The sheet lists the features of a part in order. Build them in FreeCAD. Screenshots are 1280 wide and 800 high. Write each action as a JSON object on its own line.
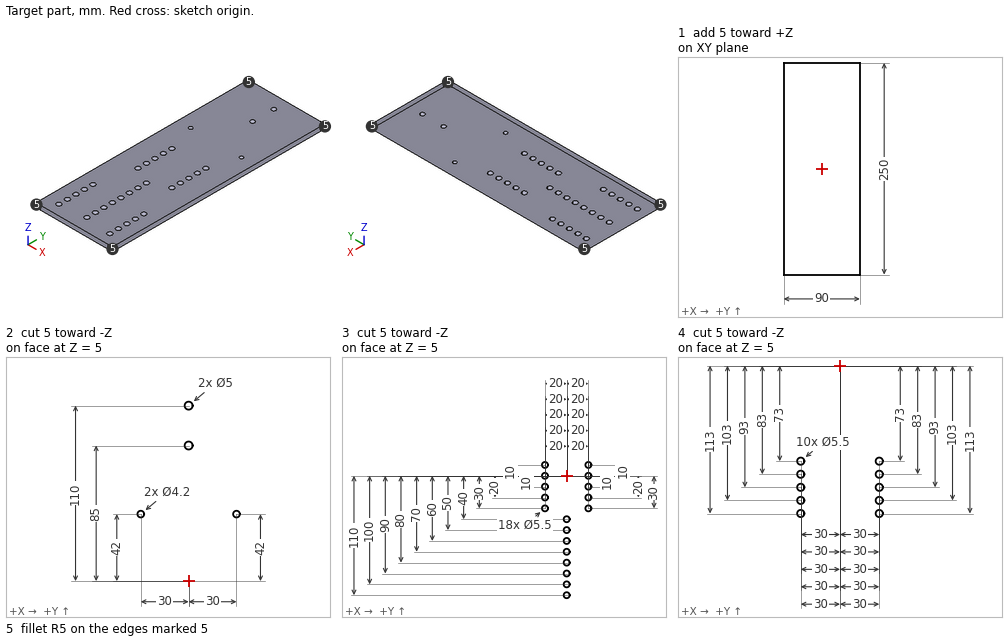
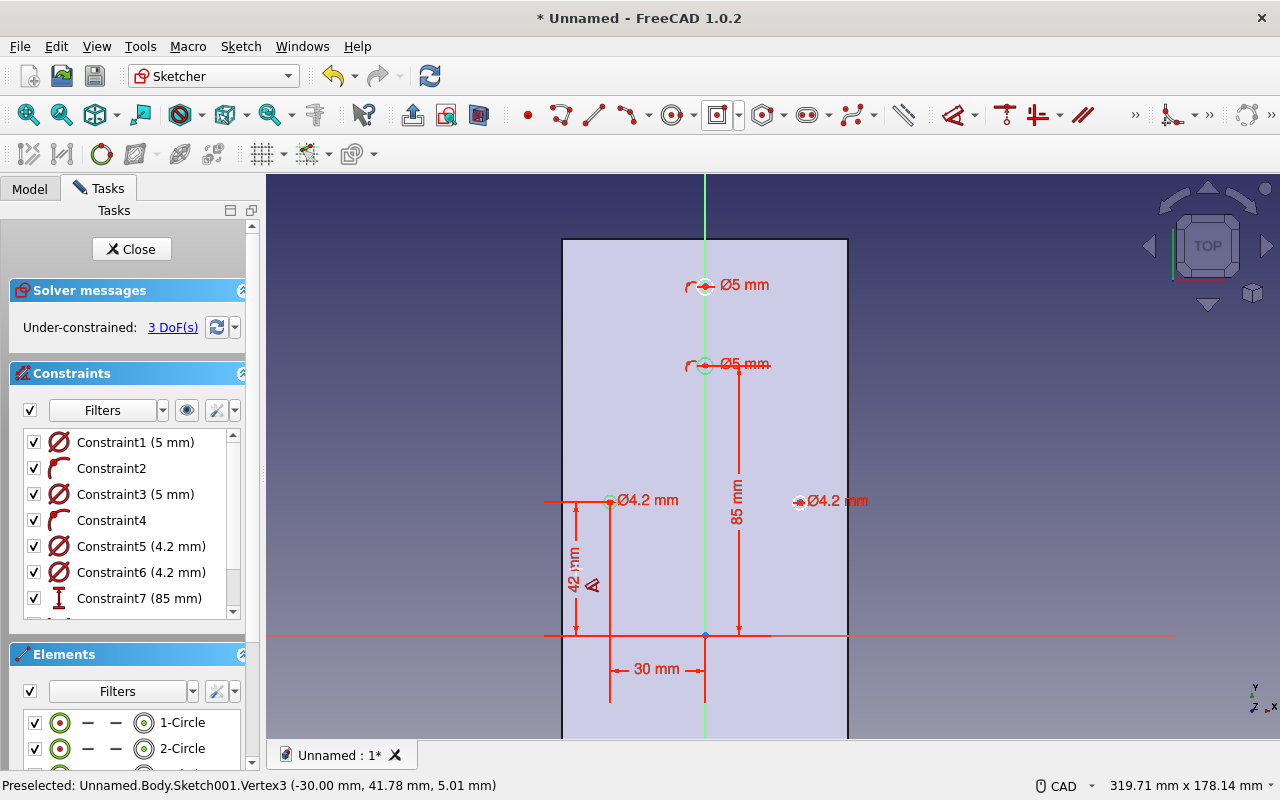
{"action": "left_click", "coordinate": [800, 503]}
{"action": "left_click", "coordinate": [753, 670]}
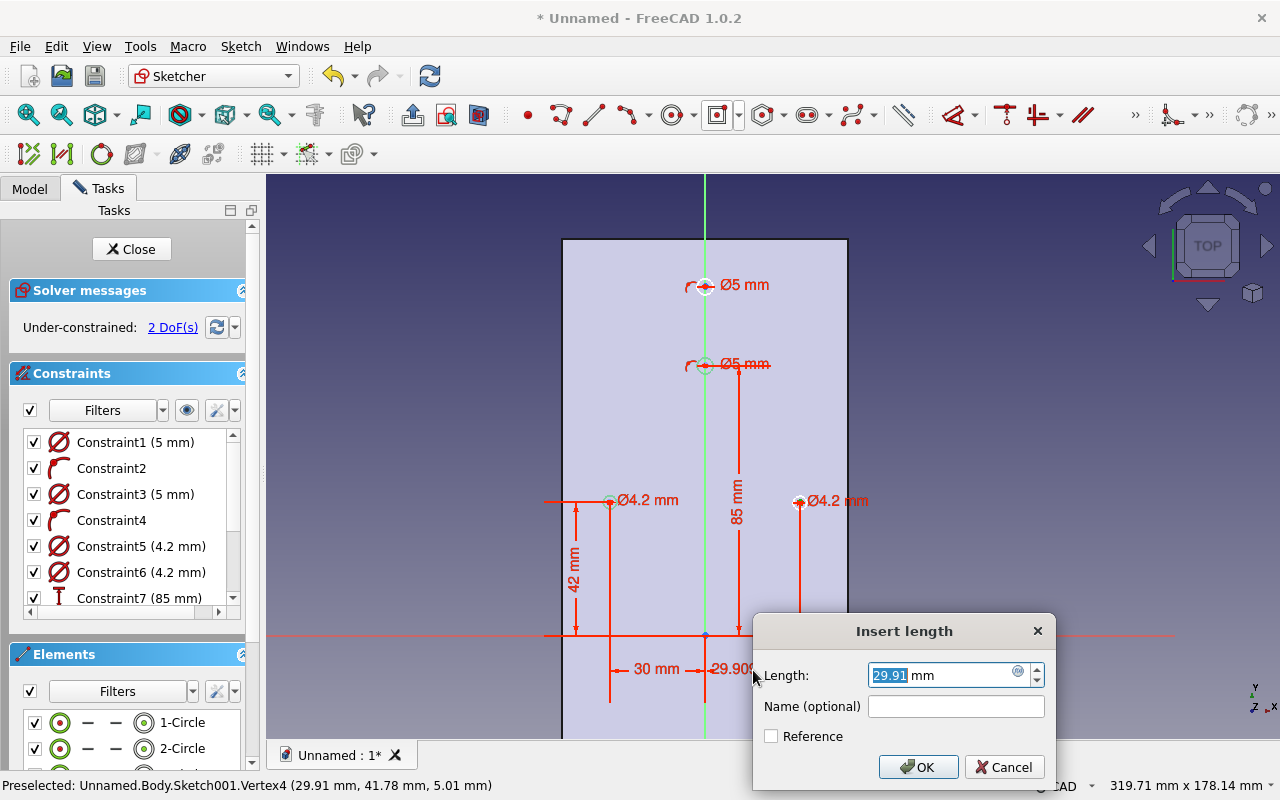
{"action": "type", "text": "30"}
{"action": "key", "text": "Return"}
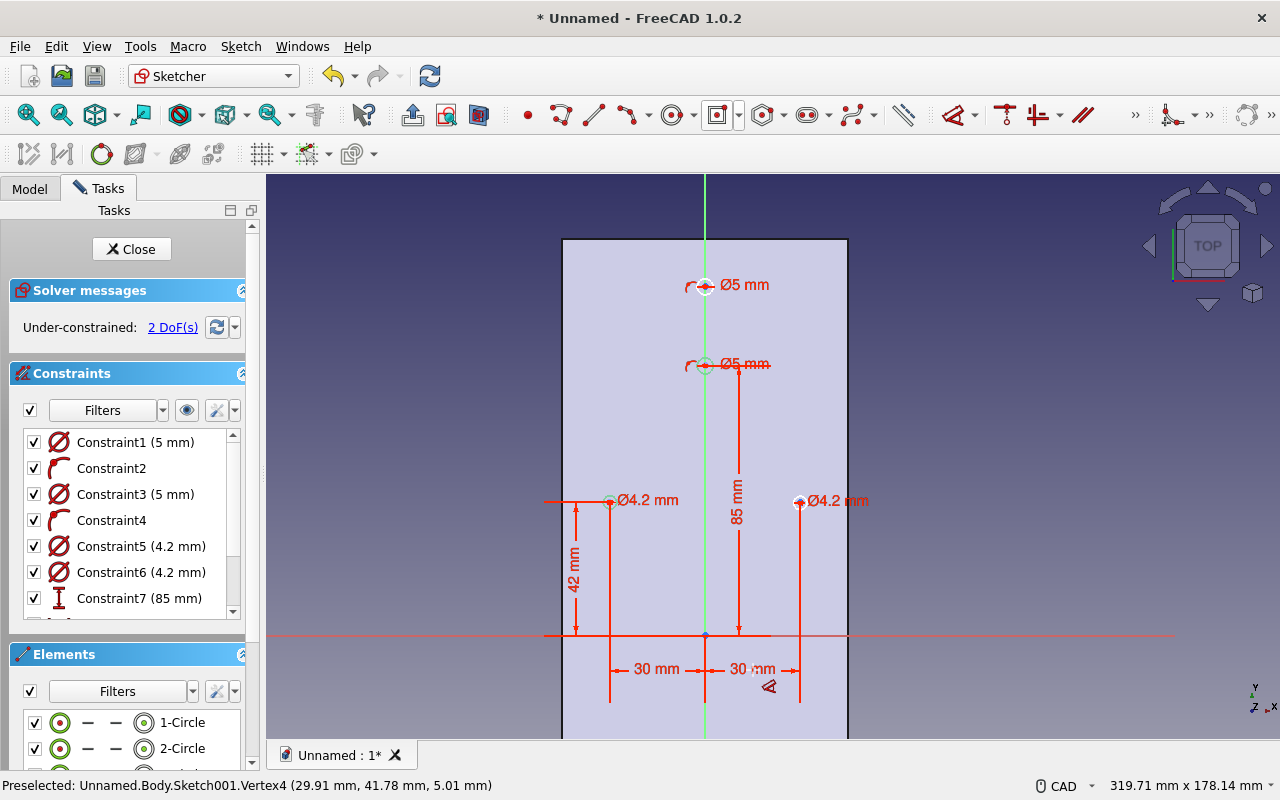
{"action": "left_click", "coordinate": [800, 503]}
{"action": "left_click", "coordinate": [834, 569]}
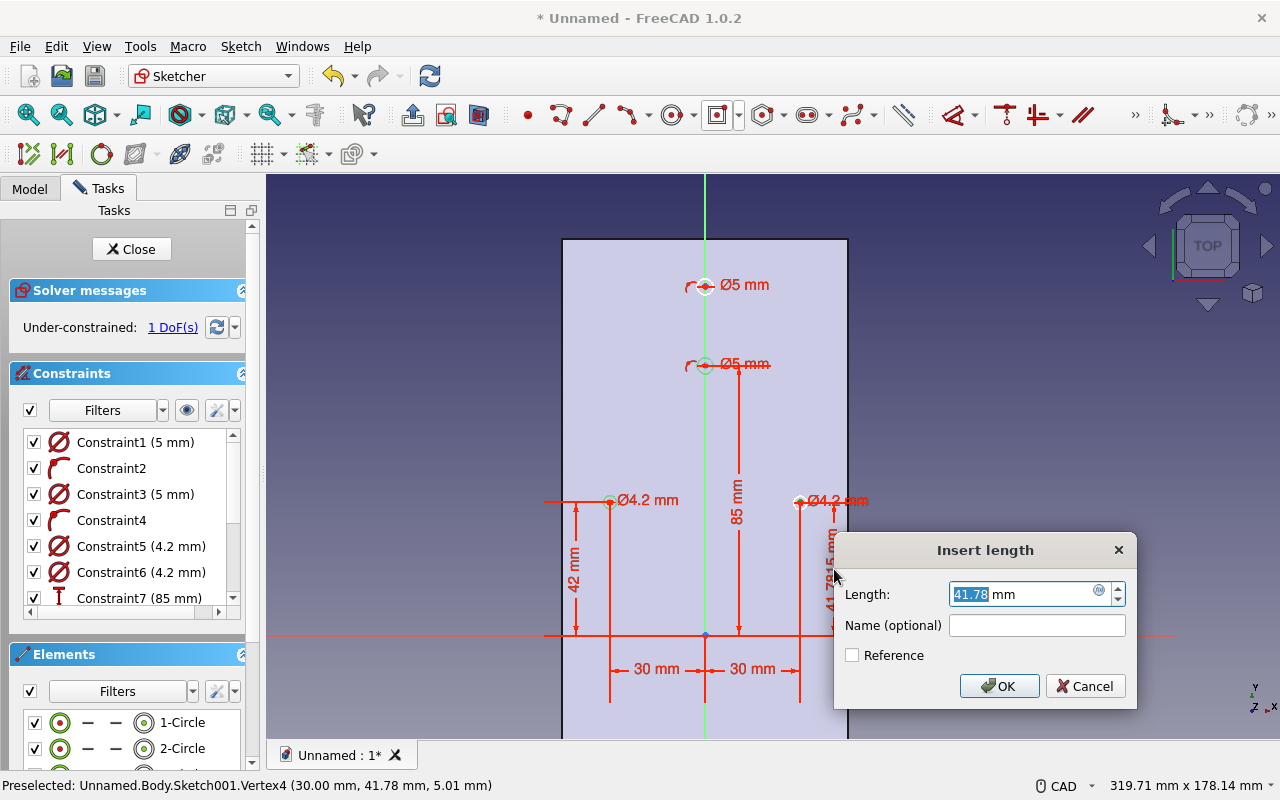
{"action": "type", "text": "42"}
{"action": "key", "text": "Return"}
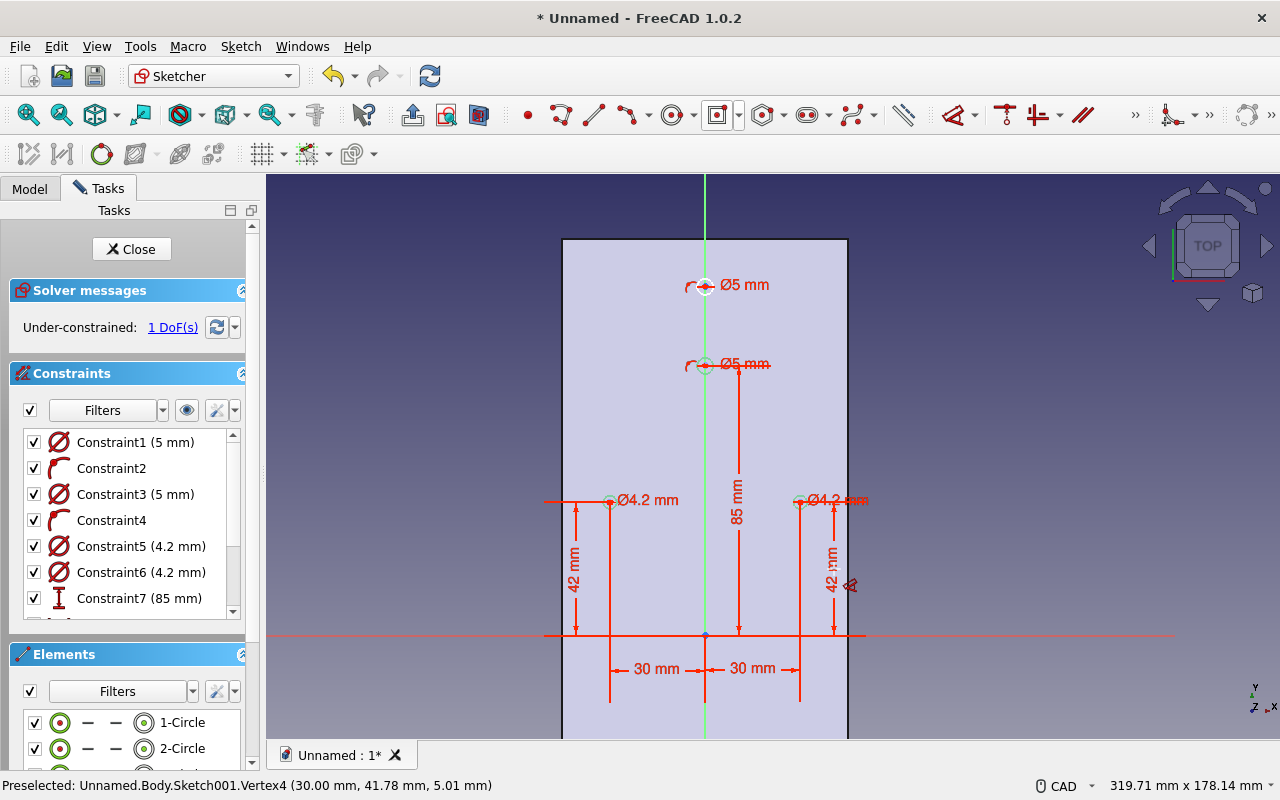
{"action": "left_click", "coordinate": [705, 287]}
{"action": "left_click", "coordinate": [739, 461]}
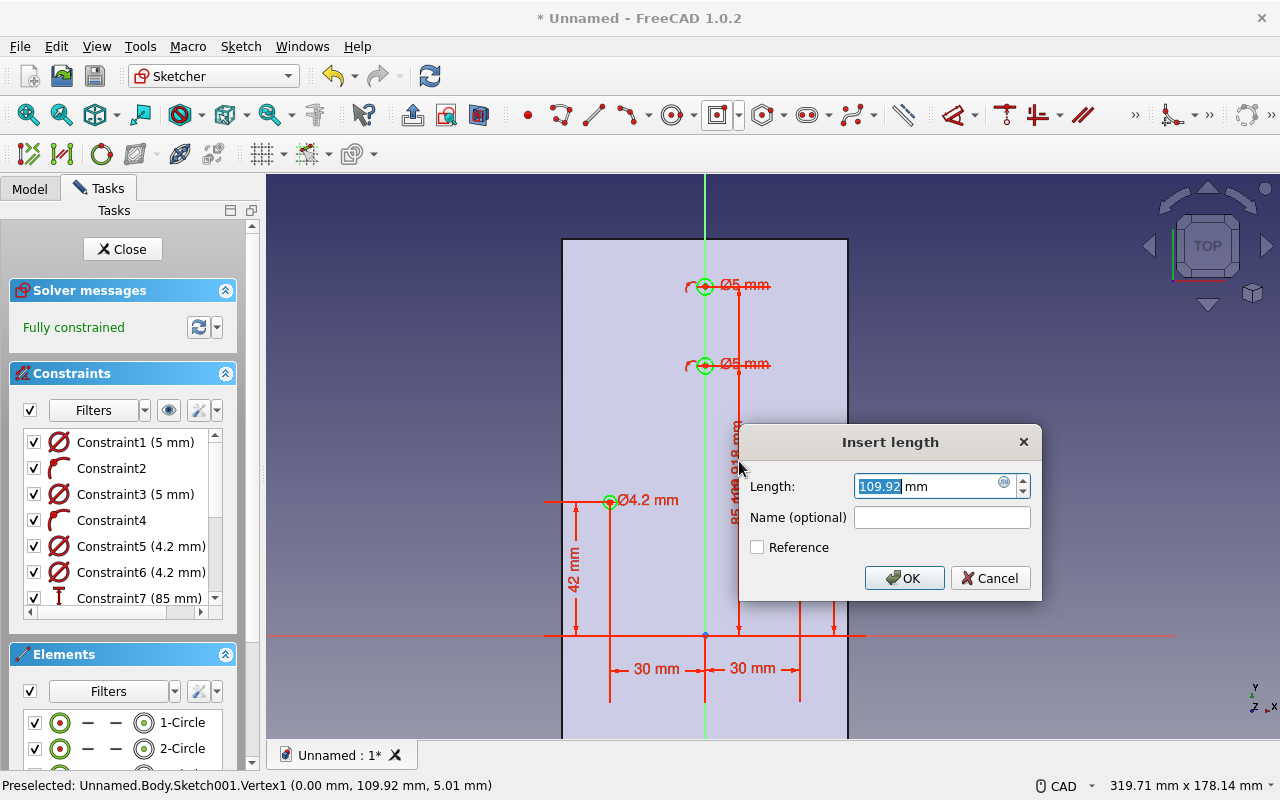
{"action": "type", "text": "110"}
{"action": "key", "text": "Return"}
{"action": "key", "text": "Escape"}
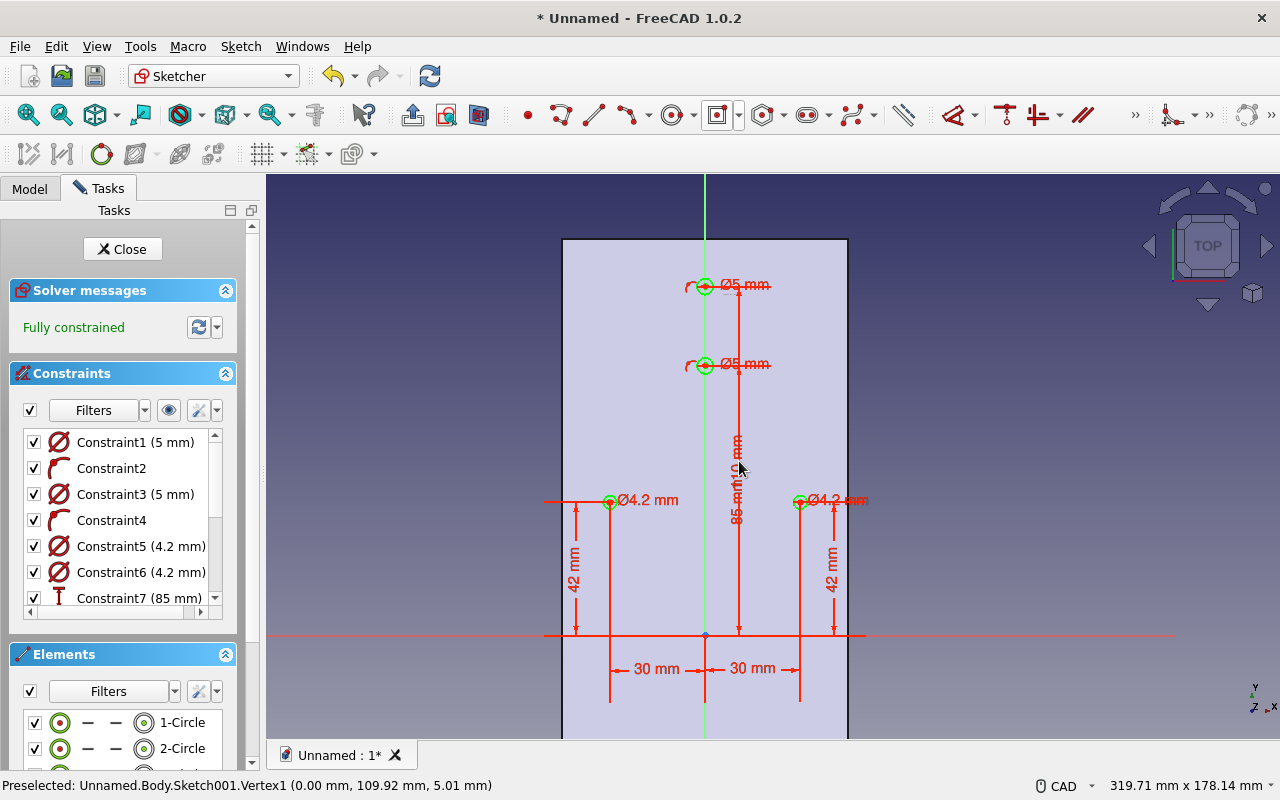
{"action": "left_click", "coordinate": [123, 249]}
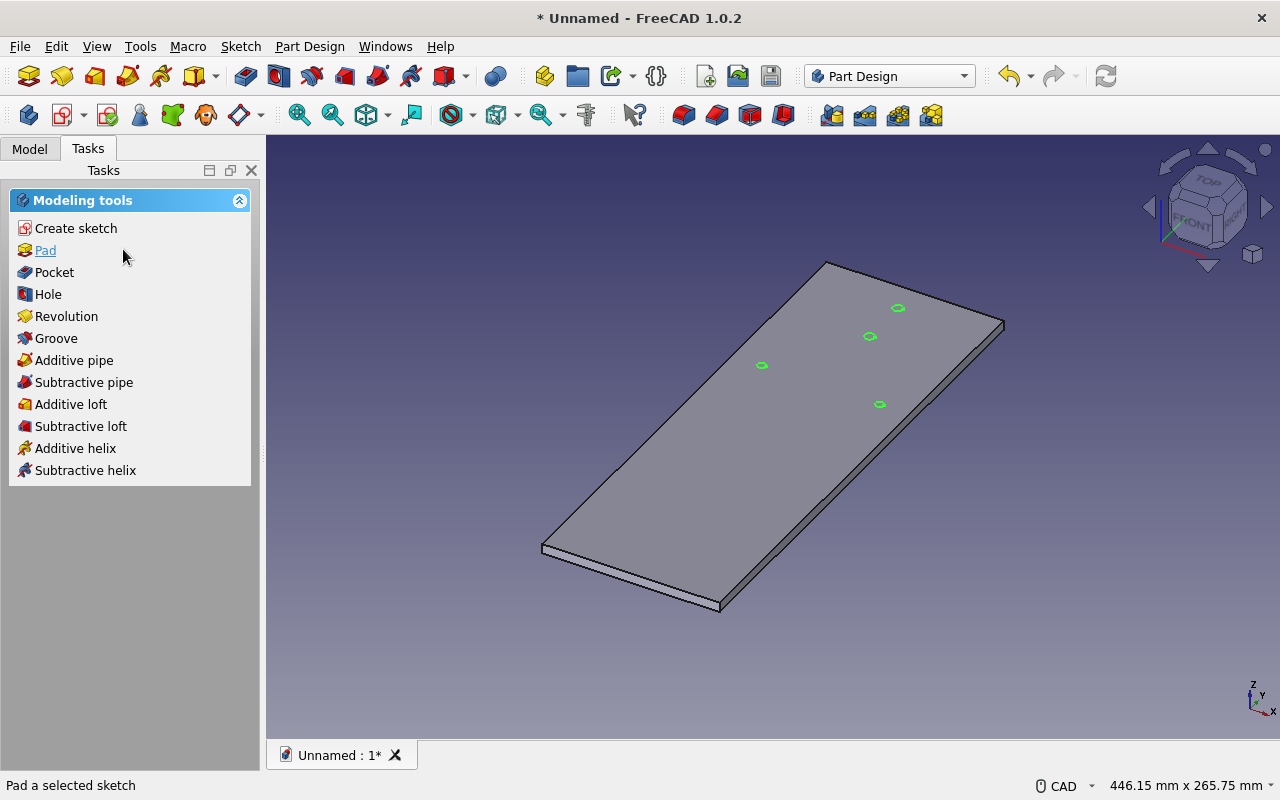
{"action": "left_click", "coordinate": [246, 76]}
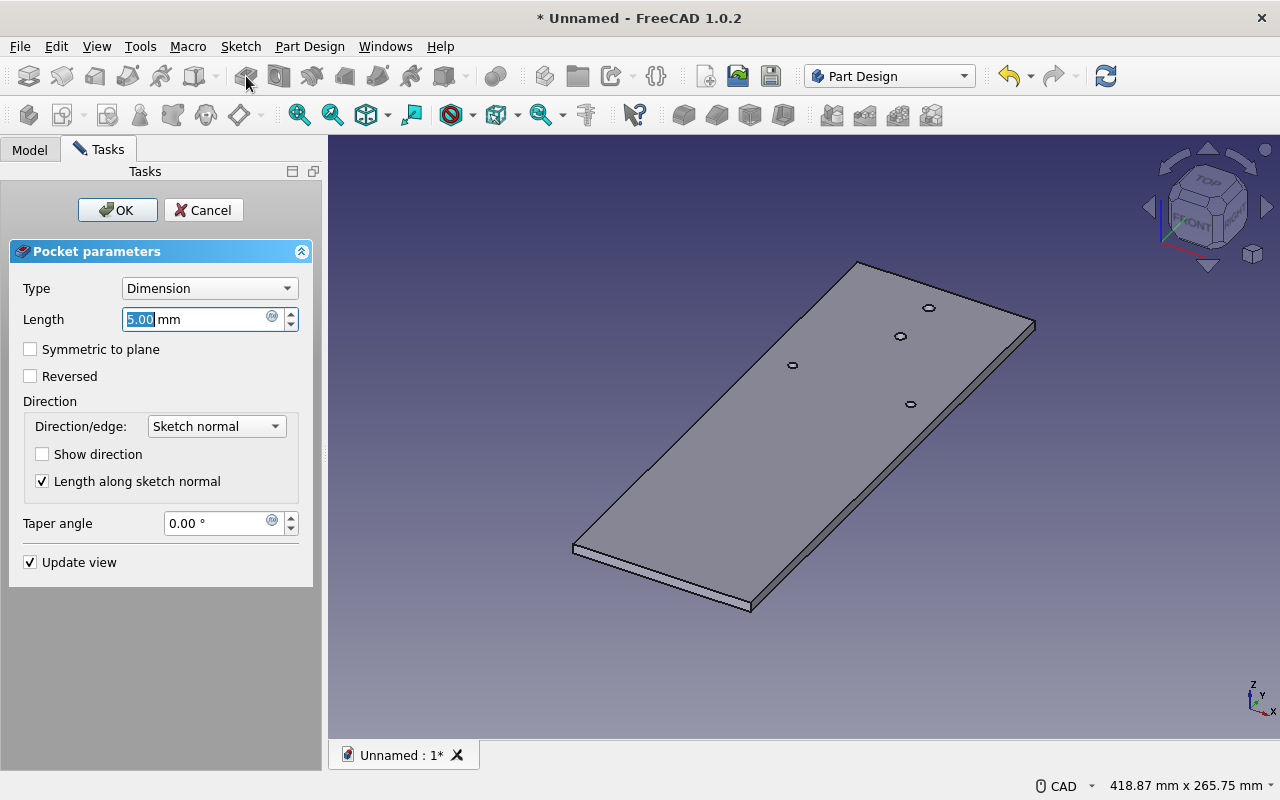
{"action": "type", "text": "5"}
{"action": "key", "text": "Tab"}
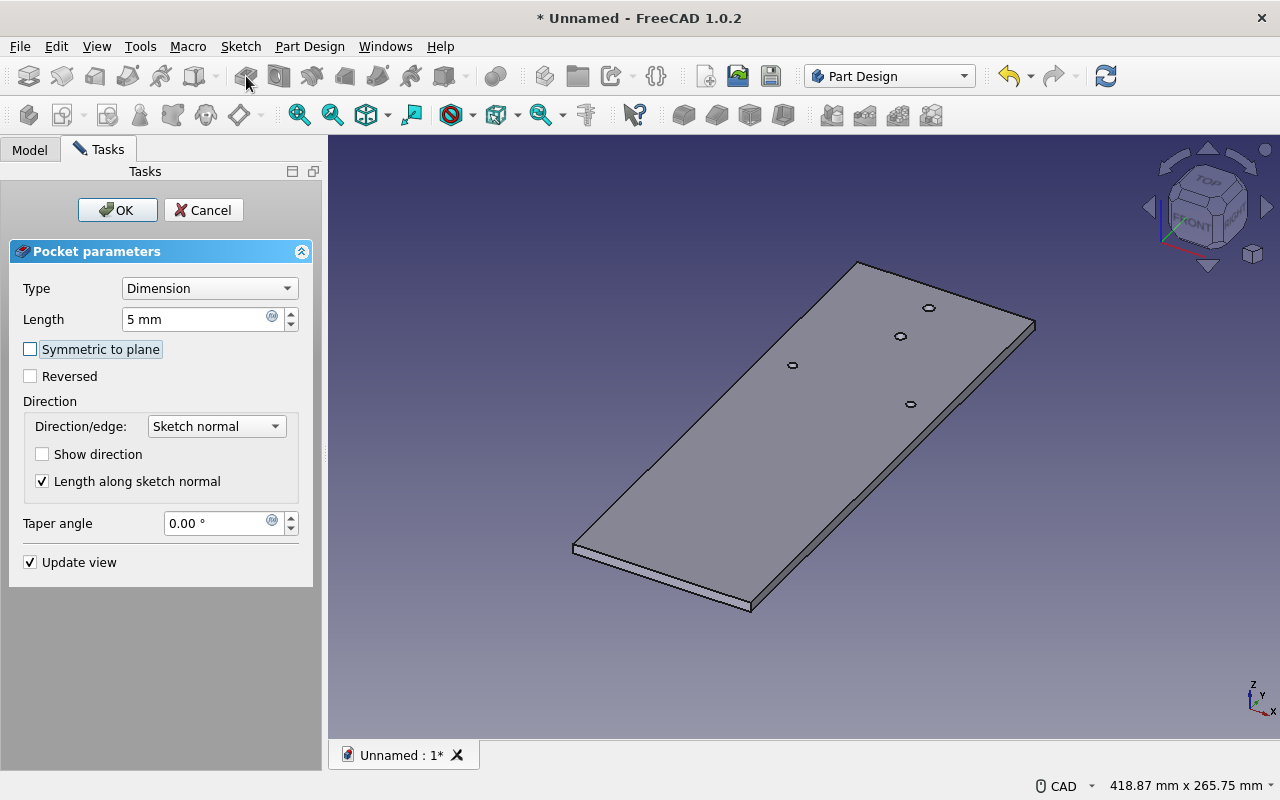
{"action": "left_click", "coordinate": [118, 210]}